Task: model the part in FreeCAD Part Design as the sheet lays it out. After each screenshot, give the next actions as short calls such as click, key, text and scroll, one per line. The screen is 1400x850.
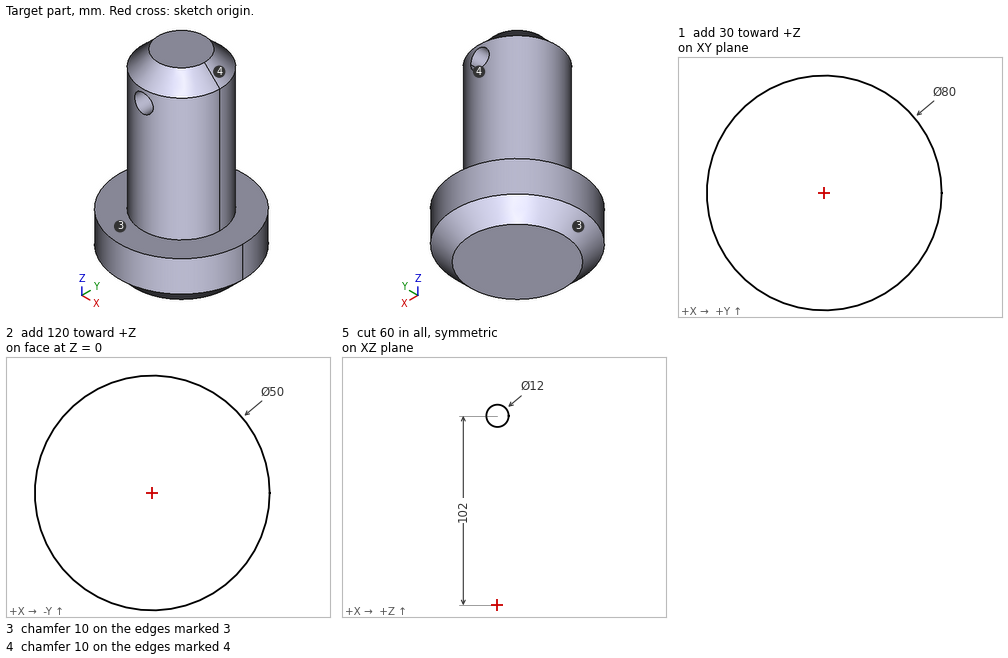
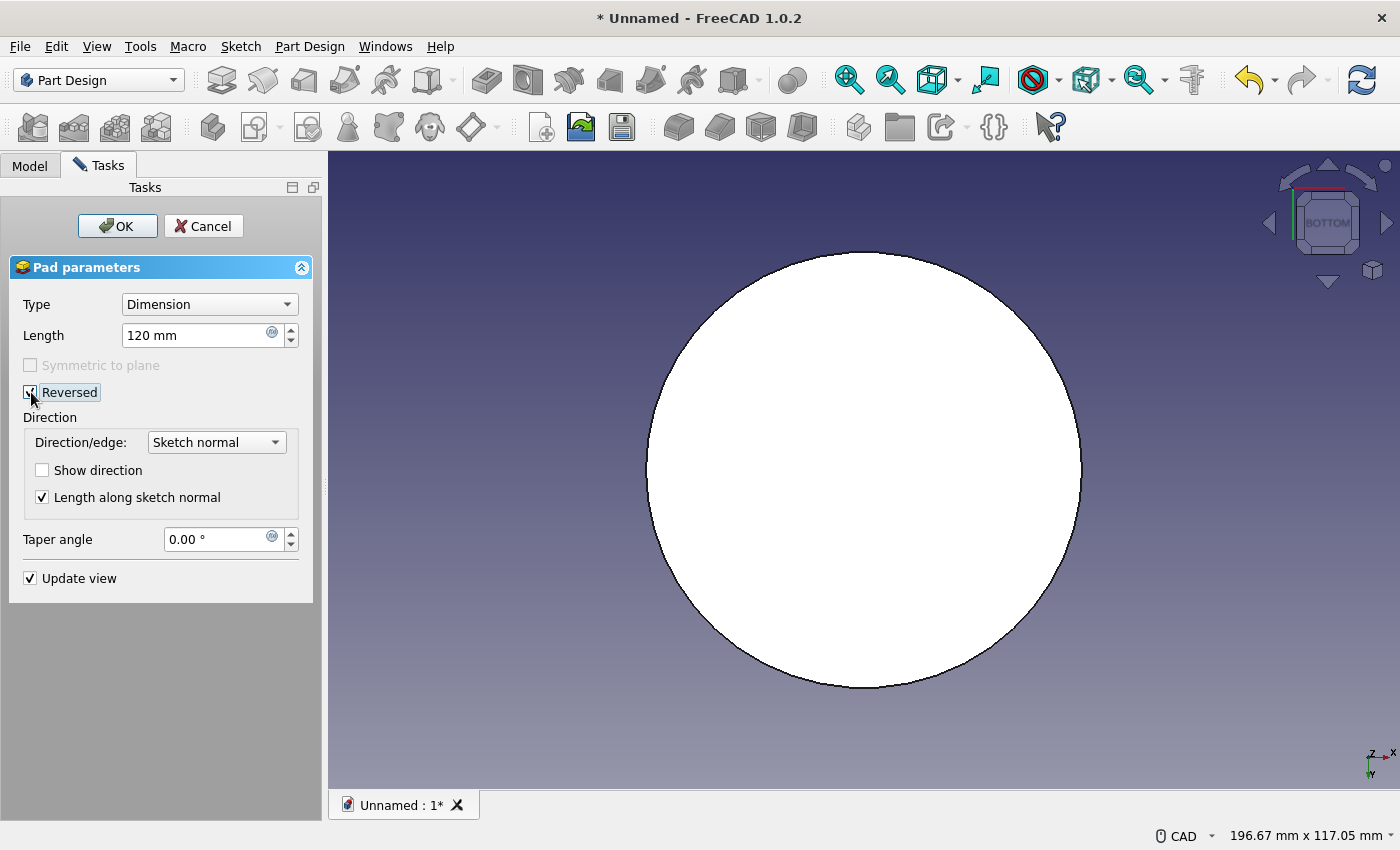
click(118, 226)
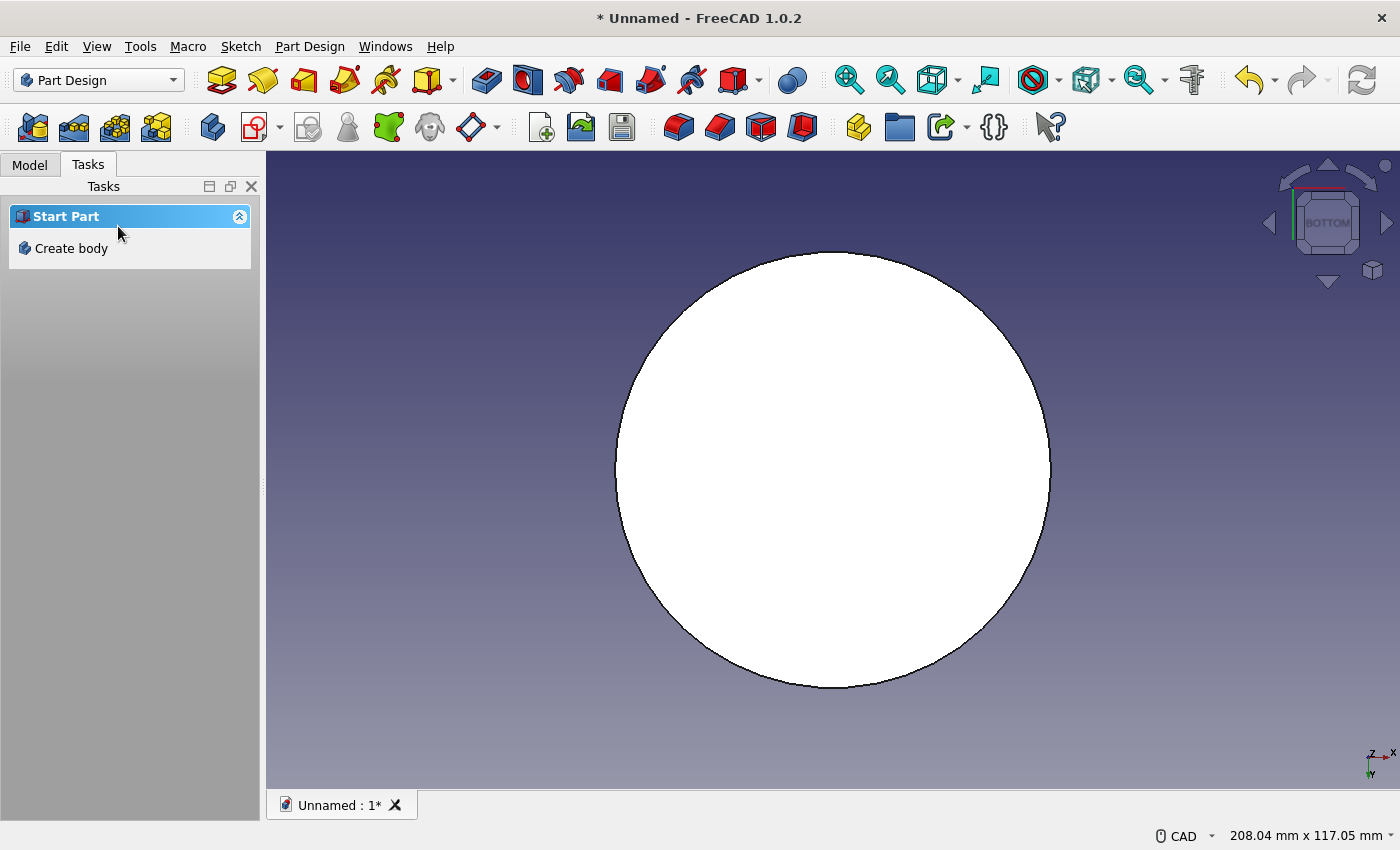
click(615, 469)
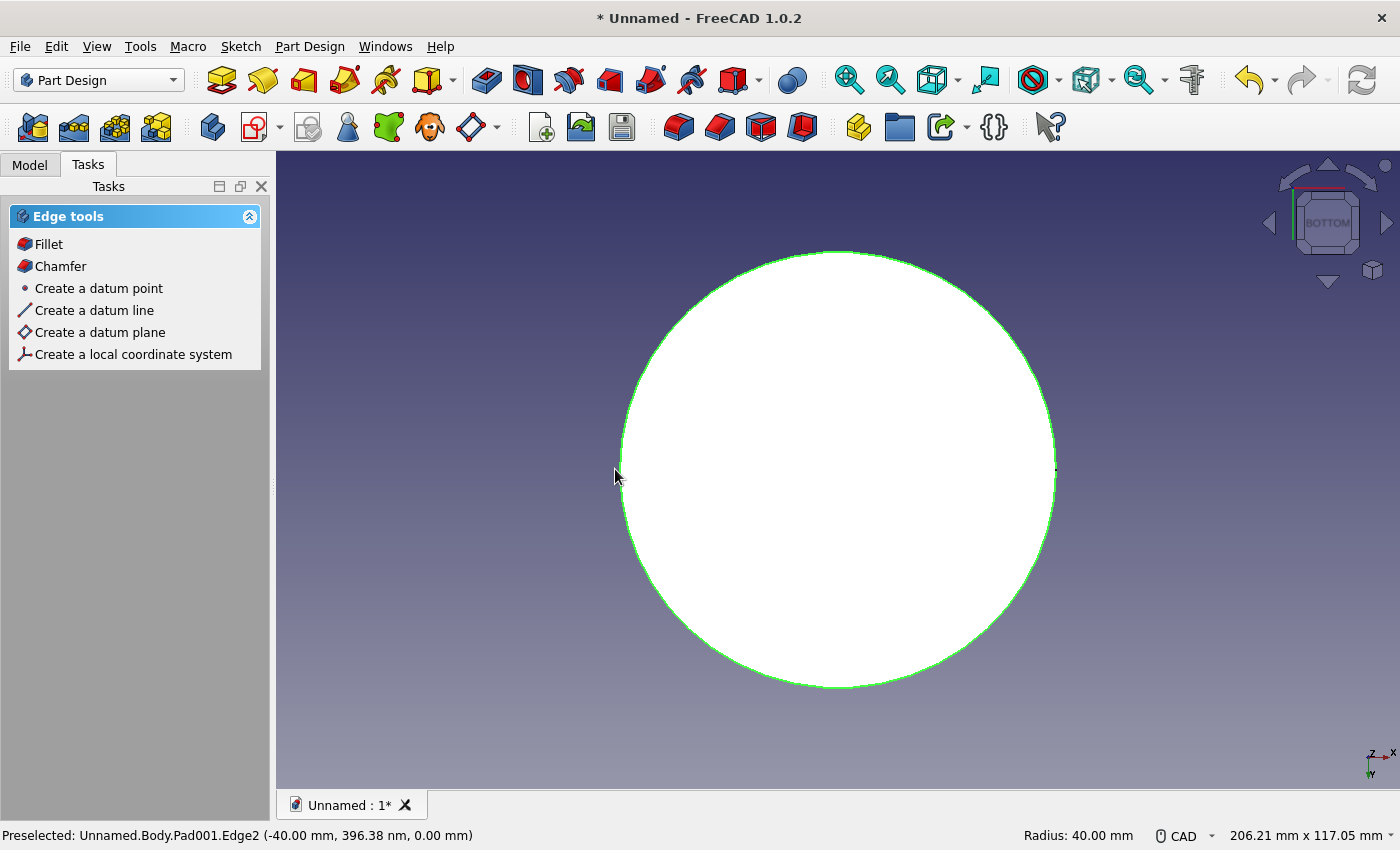
click(720, 128)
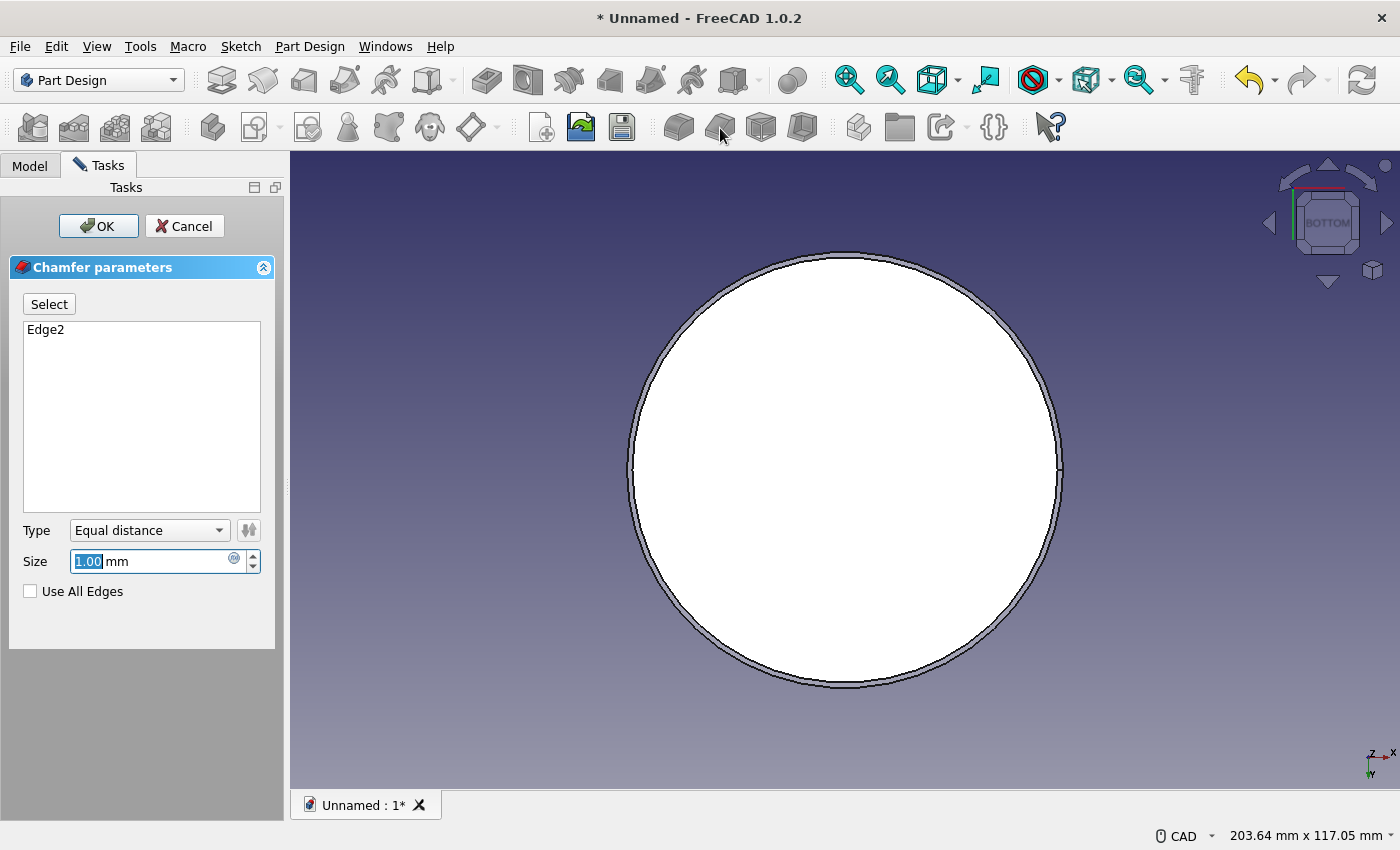
text(10)
key(Tab)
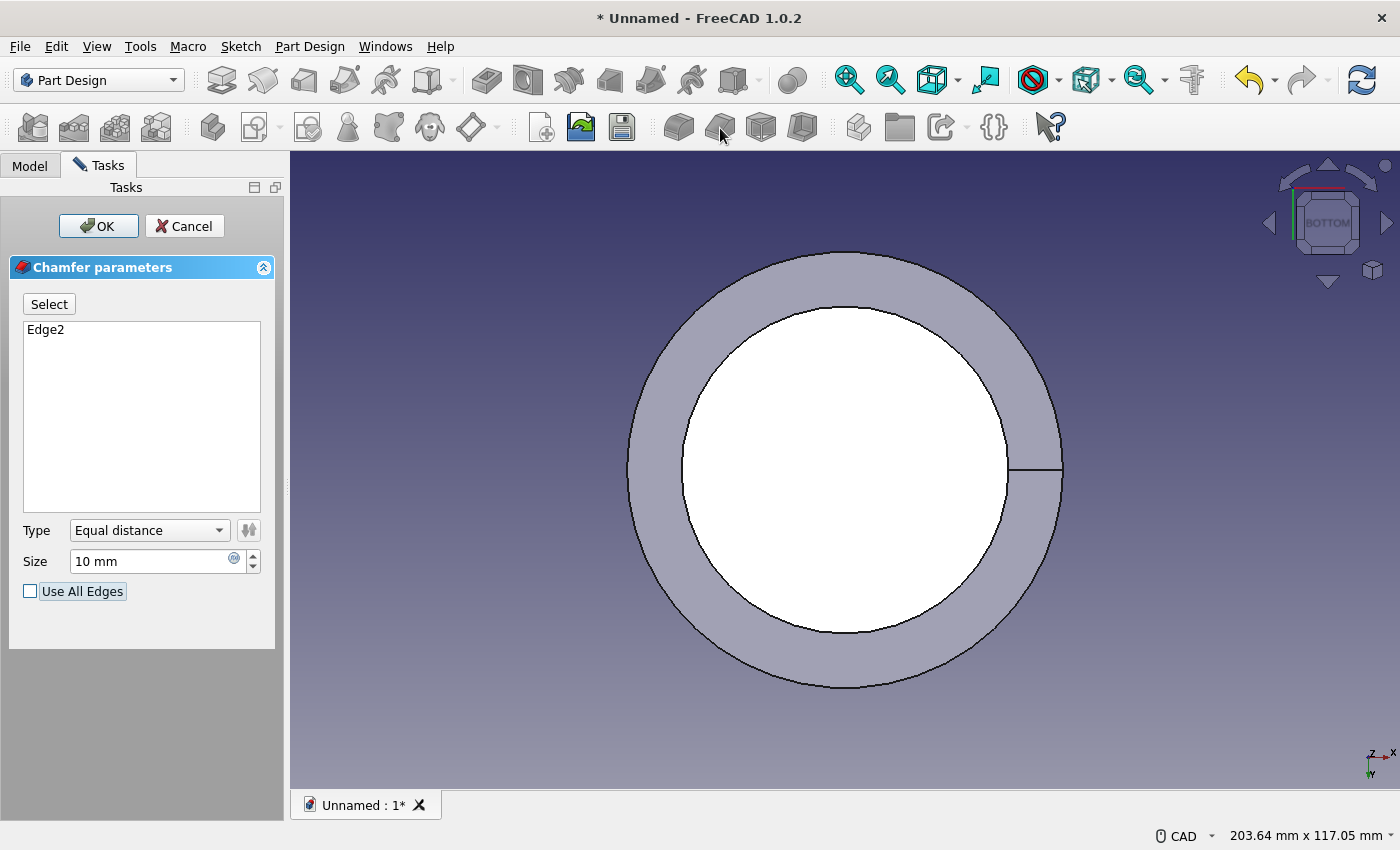
click(99, 226)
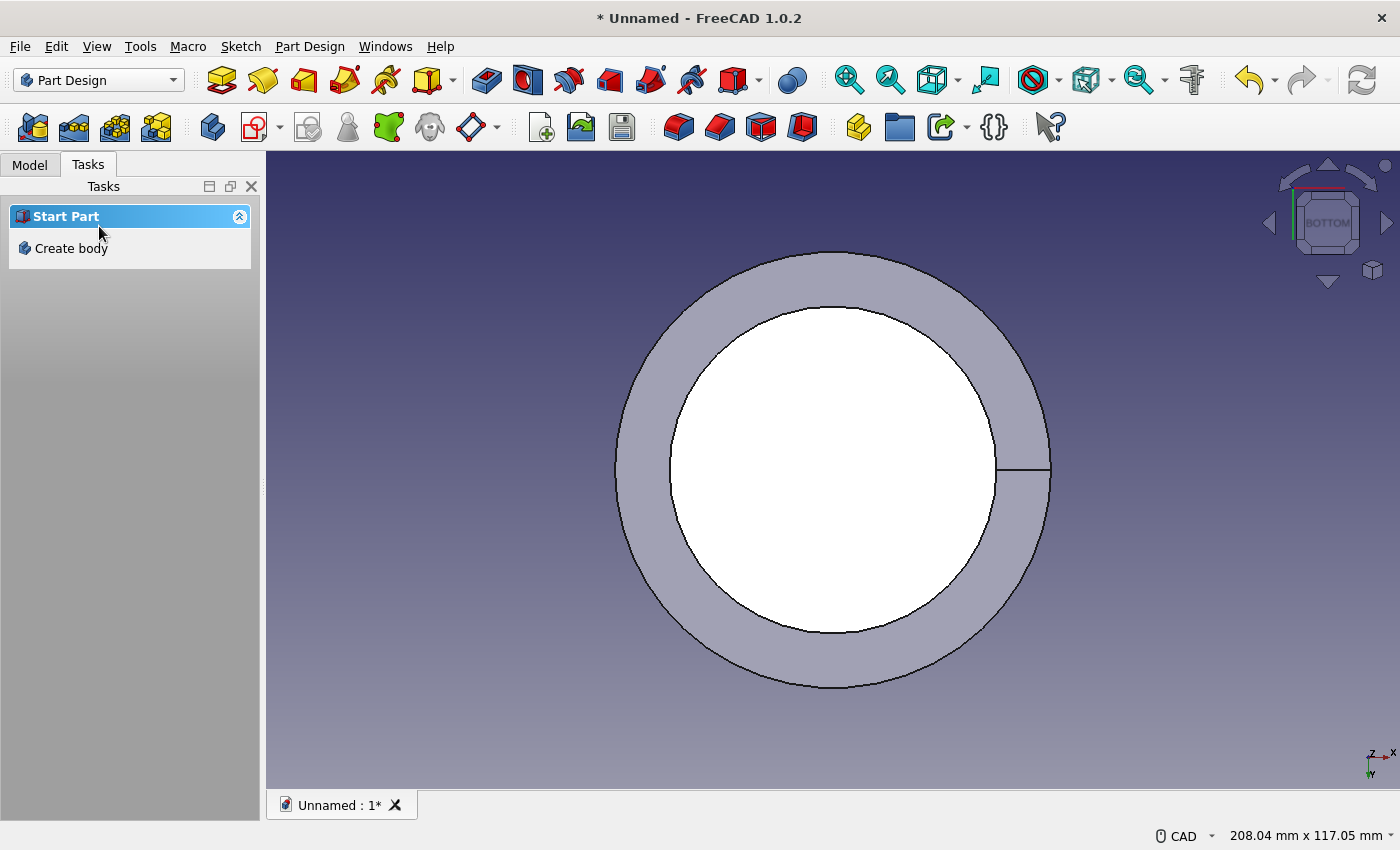
key(0)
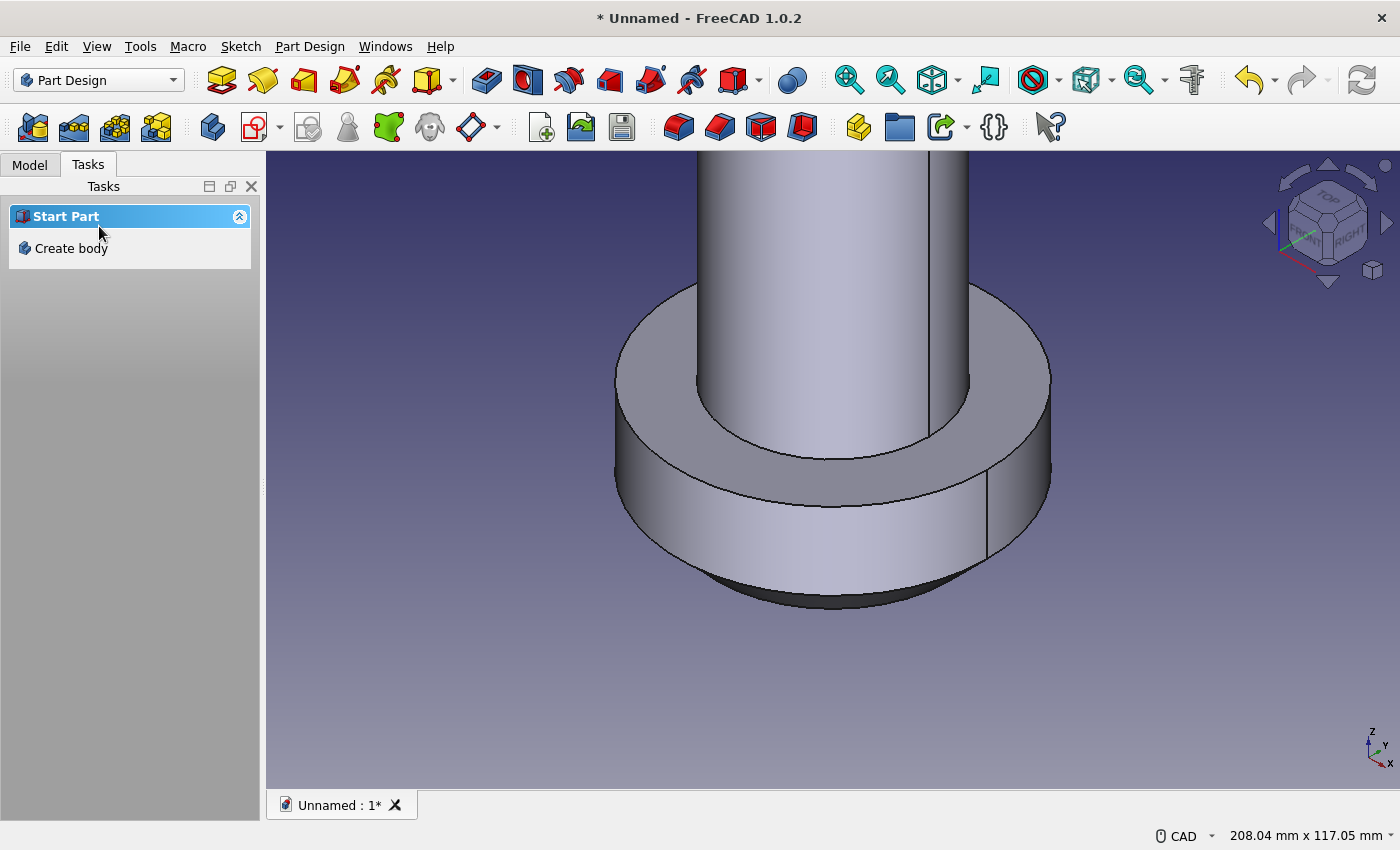
click(850, 80)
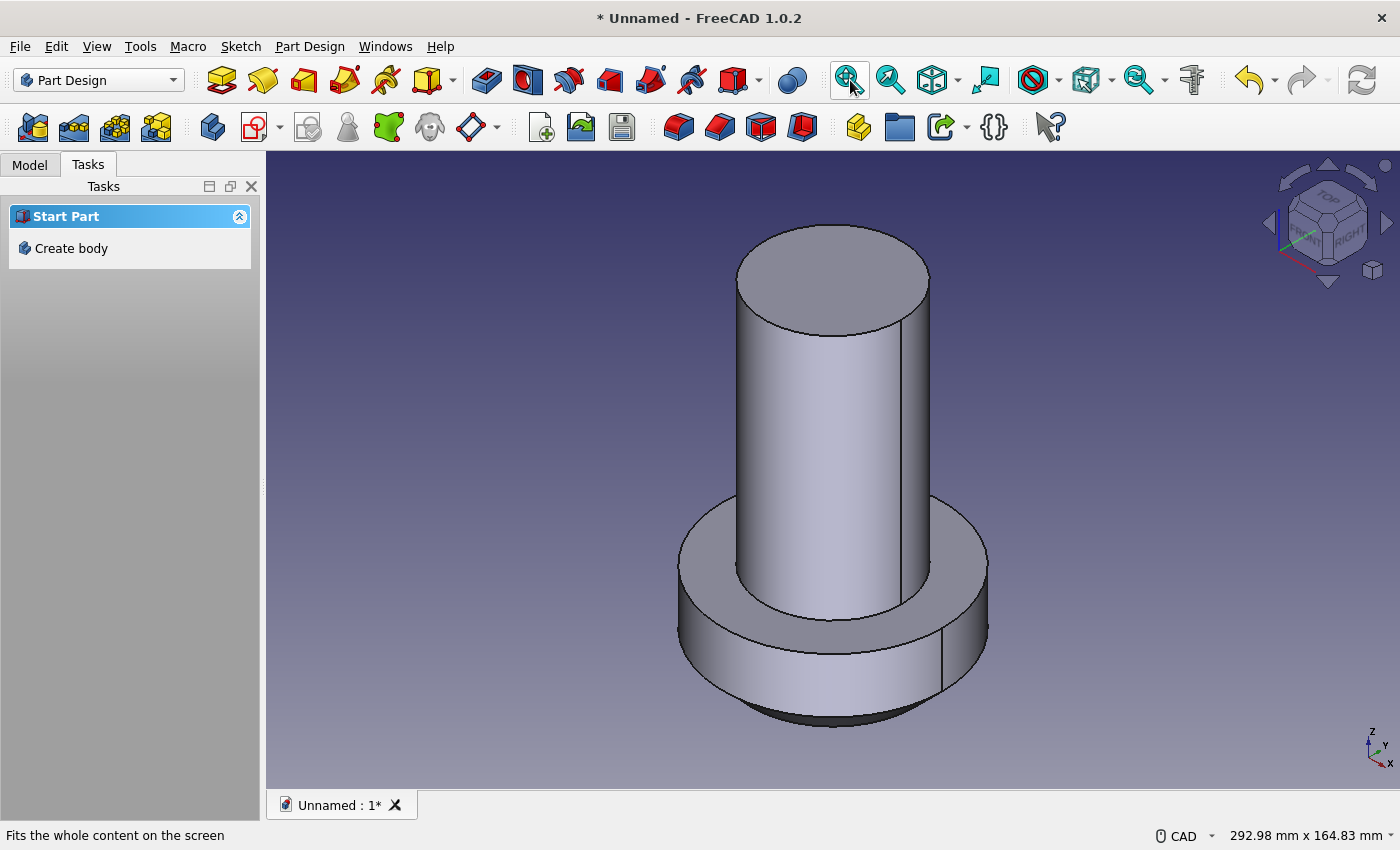
click(747, 305)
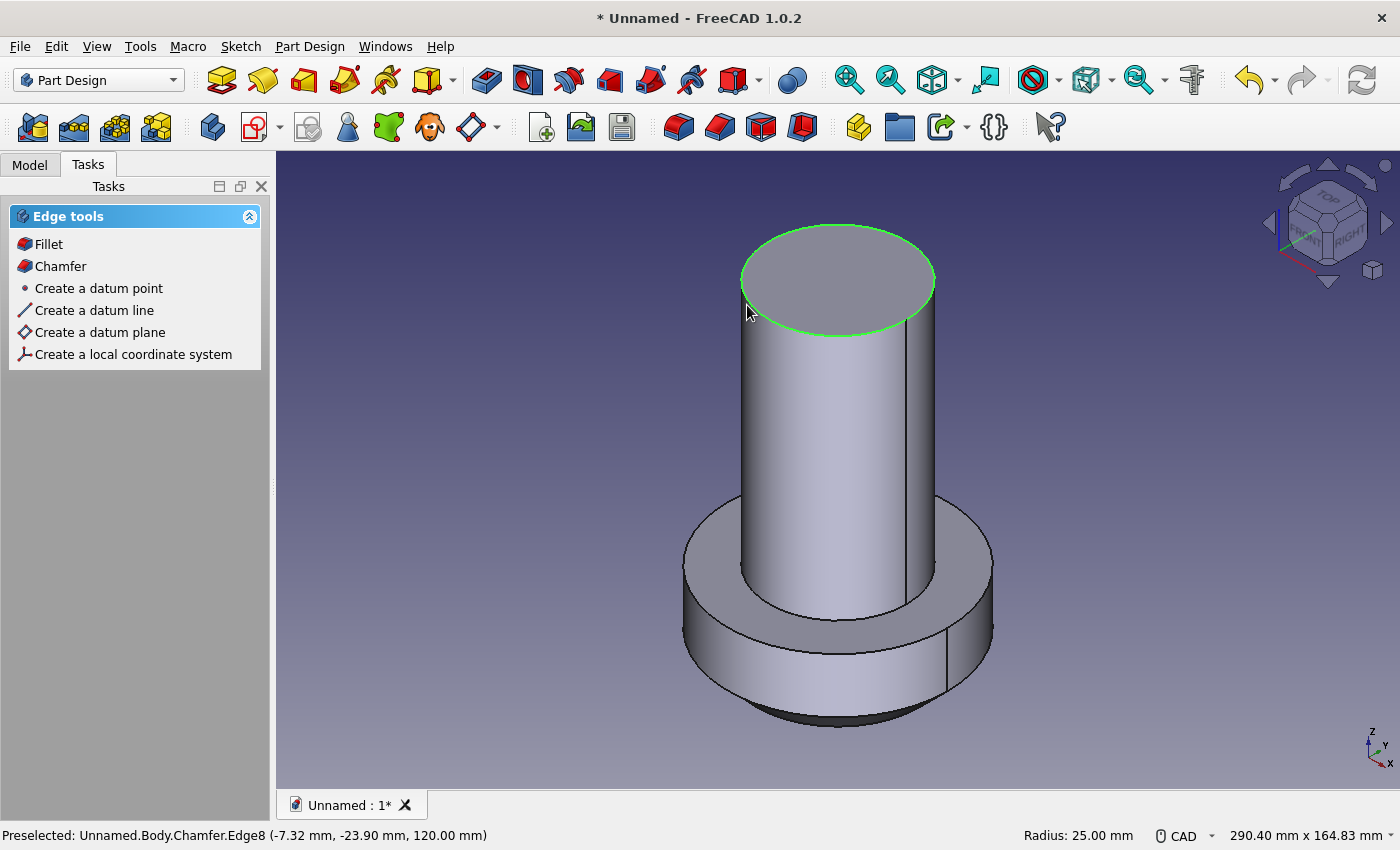
click(720, 128)